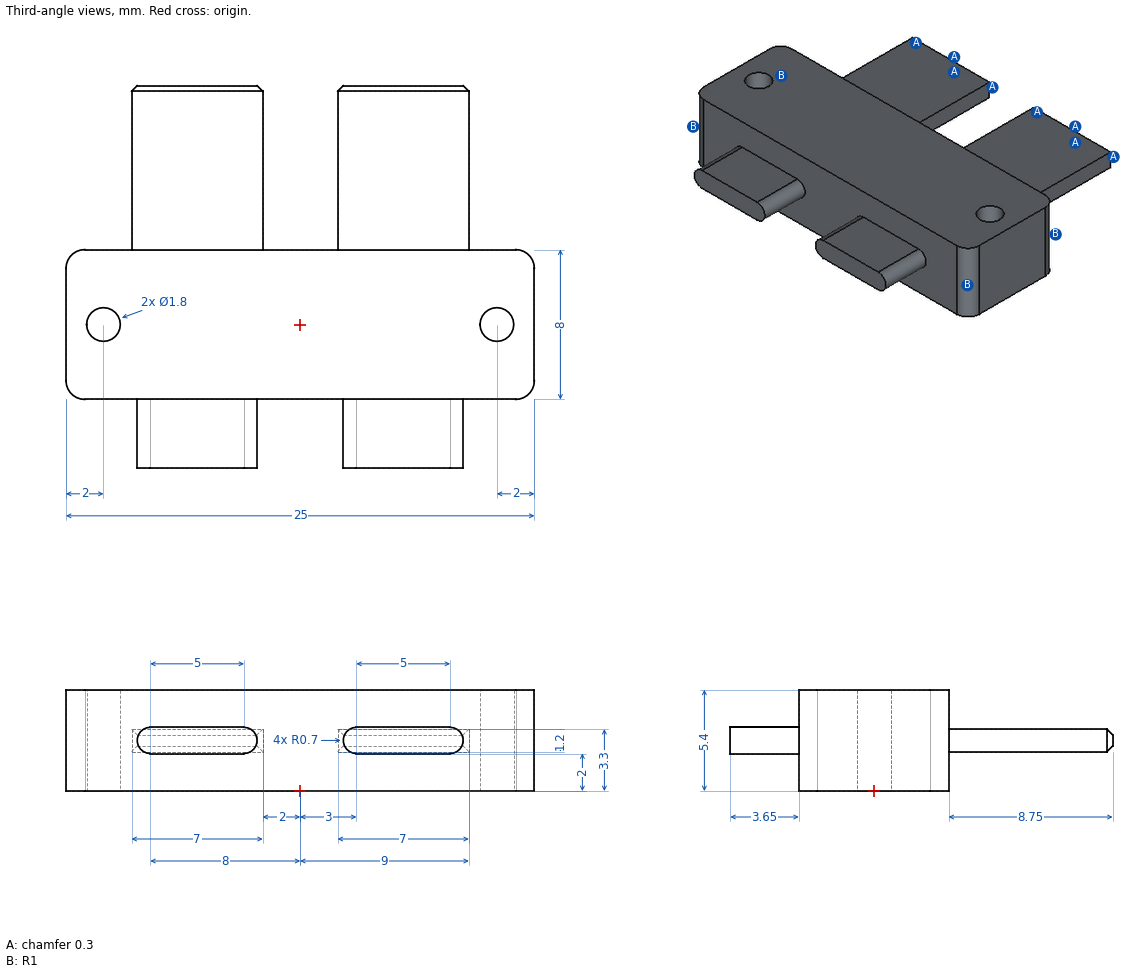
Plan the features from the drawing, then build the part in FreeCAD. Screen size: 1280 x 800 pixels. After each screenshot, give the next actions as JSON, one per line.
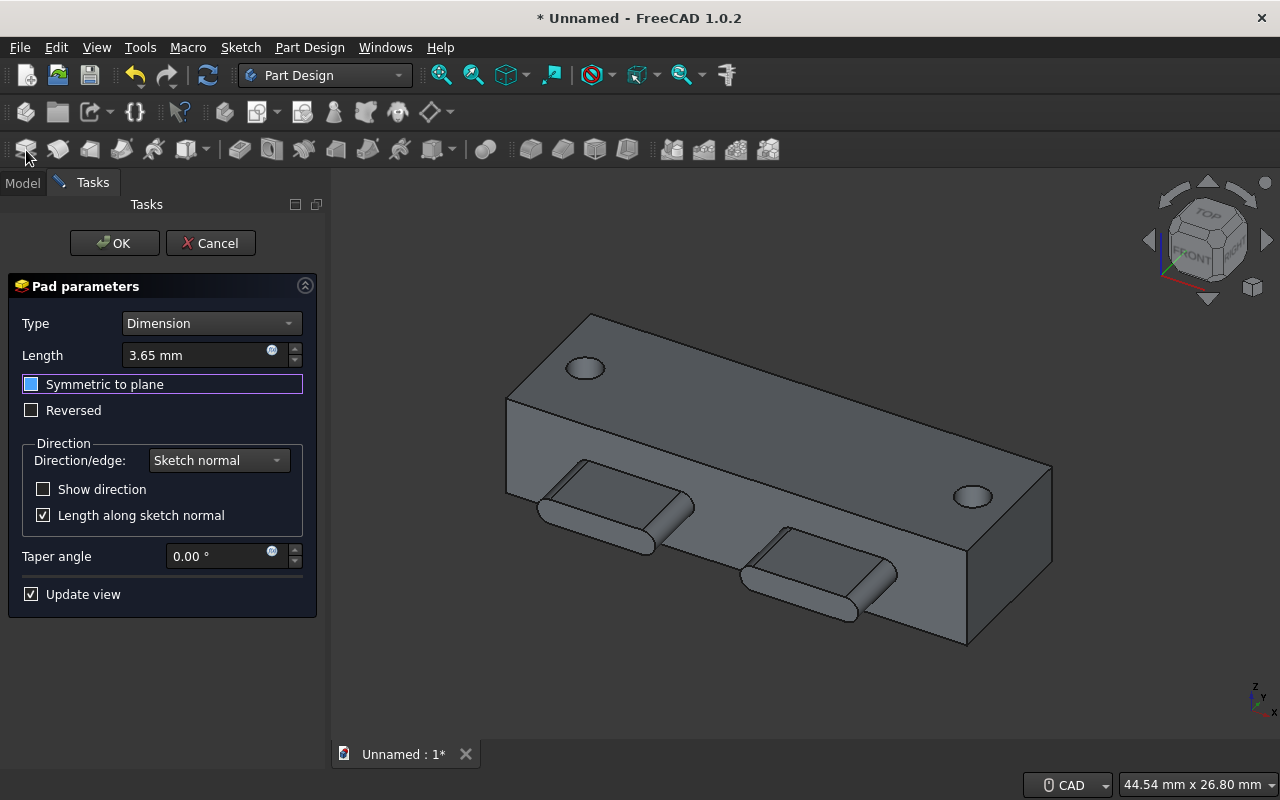
{"action": "left_click", "coordinate": [115, 243]}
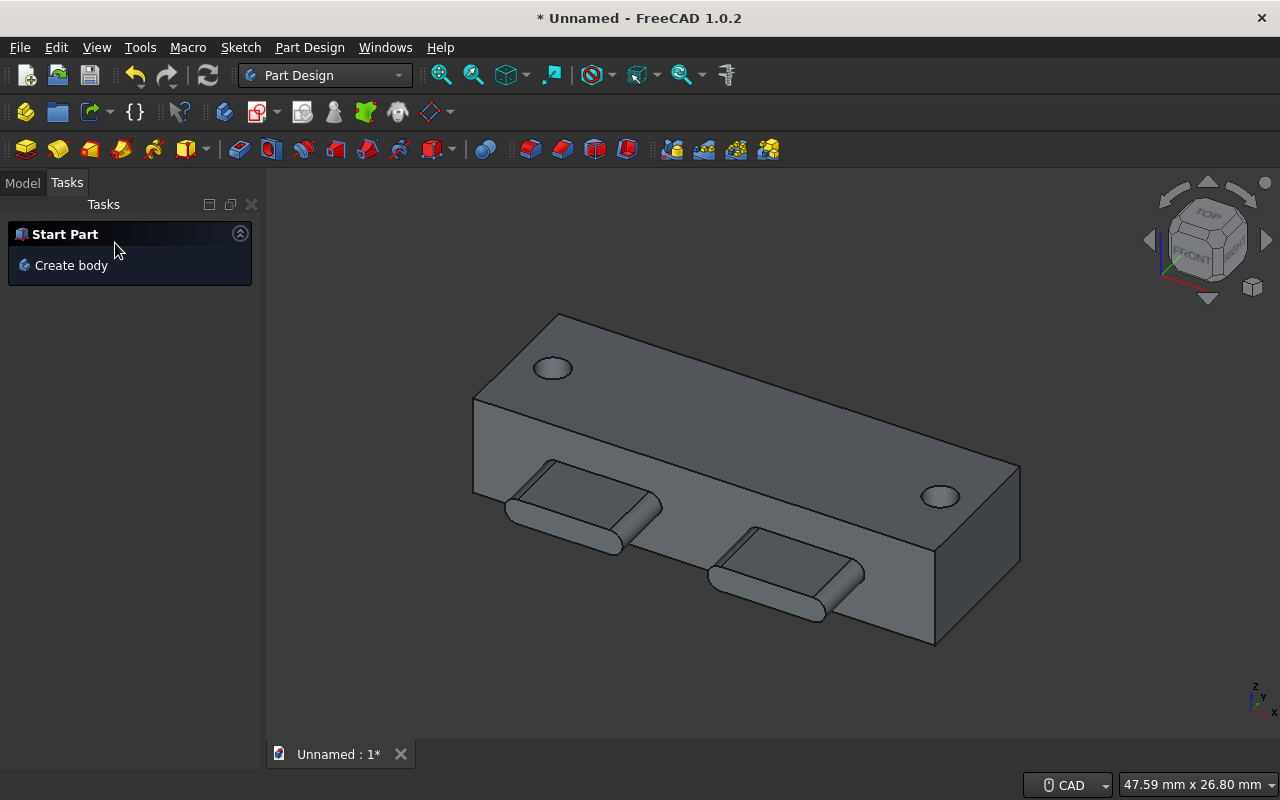
{"action": "key", "text": "4"}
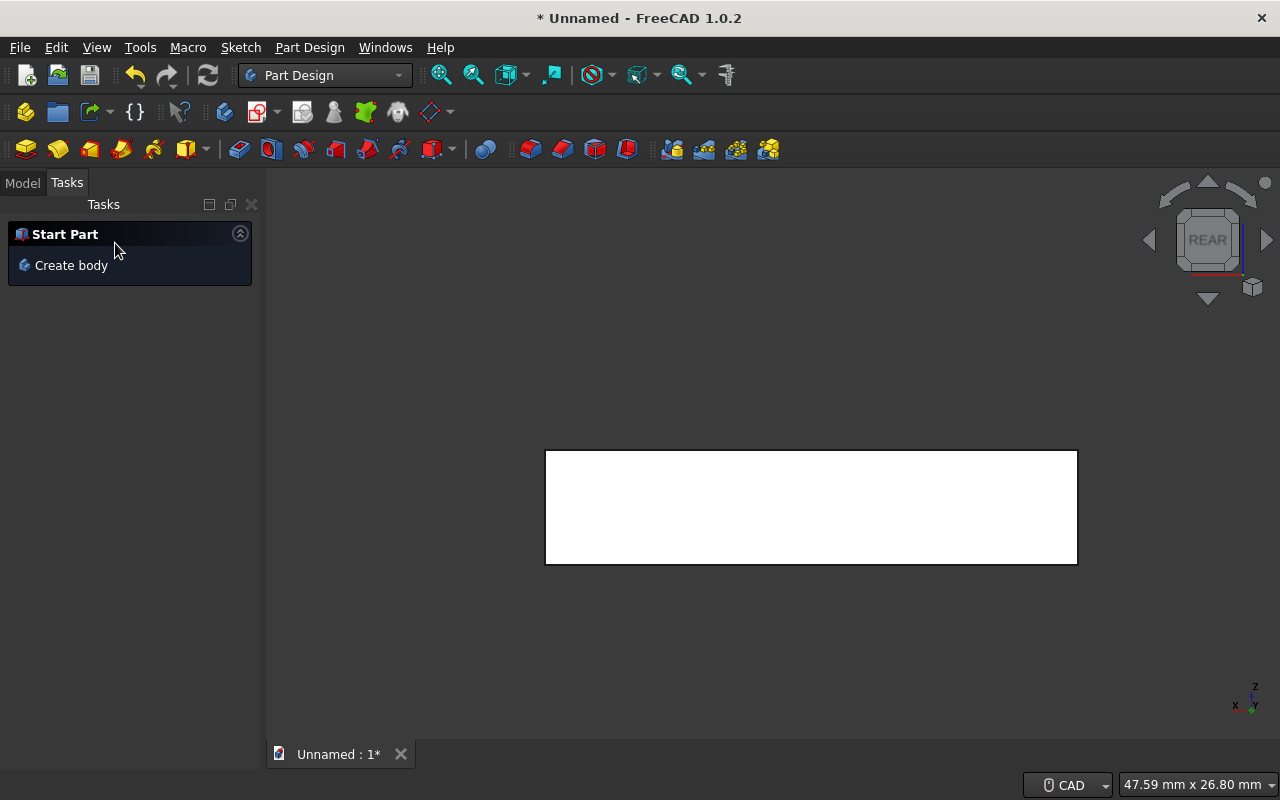
{"action": "left_click", "coordinate": [659, 506]}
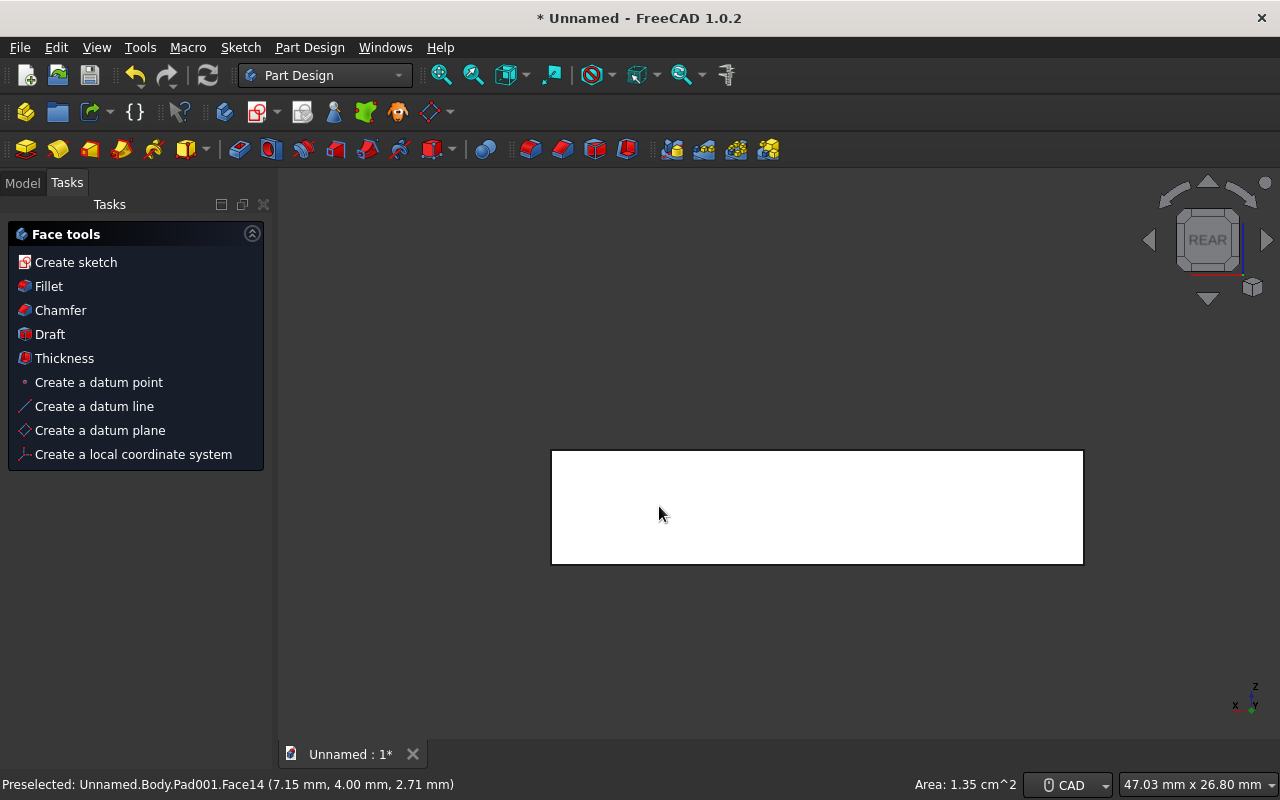
{"action": "left_click", "coordinate": [258, 112]}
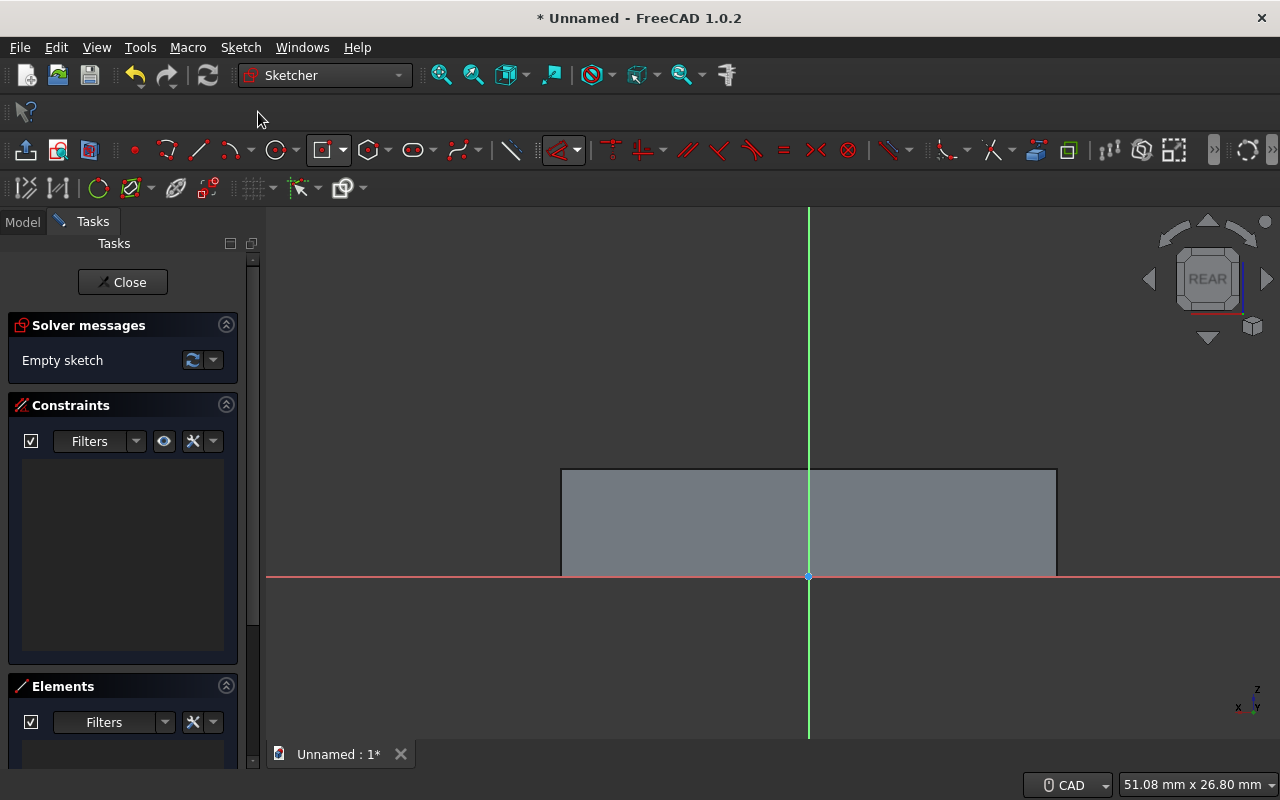
{"action": "scroll", "coordinate": [1020, 688], "scroll_direction": "up", "scroll_amount": 2}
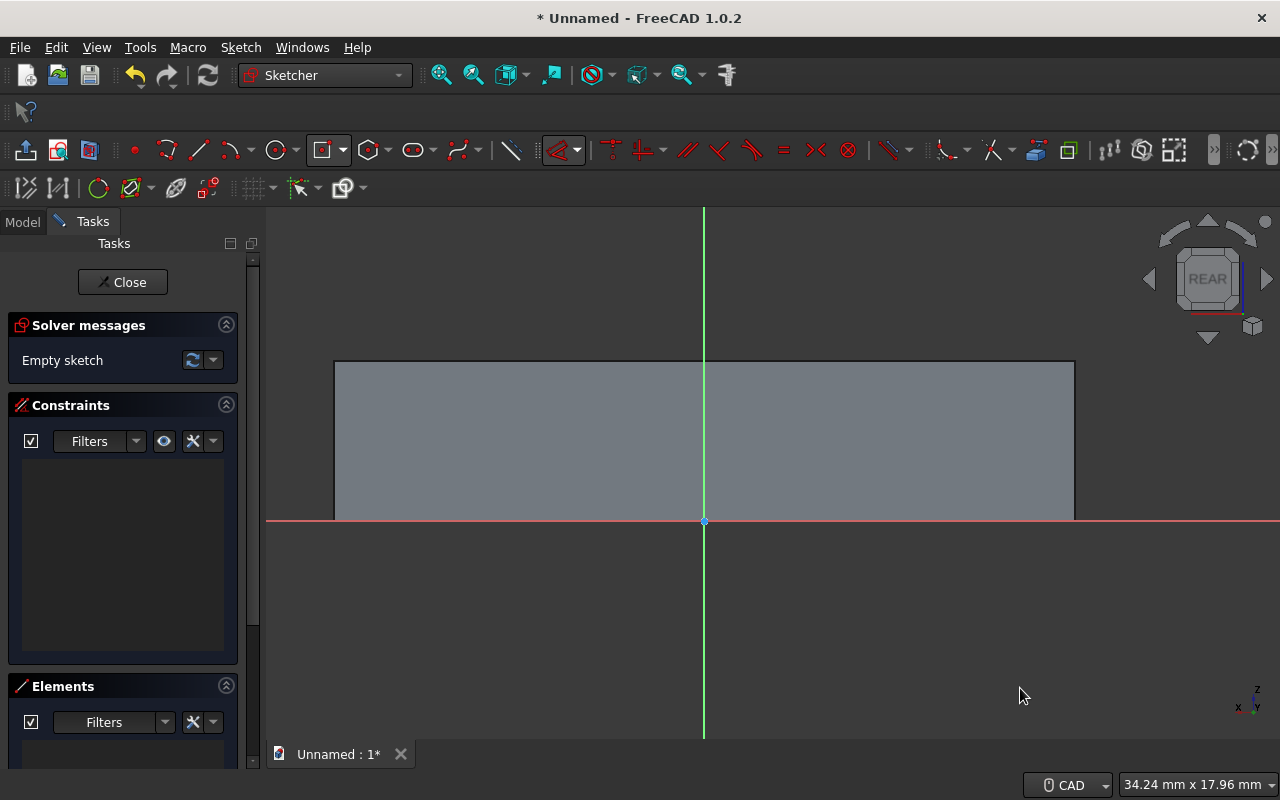
{"action": "key", "text": "g r"}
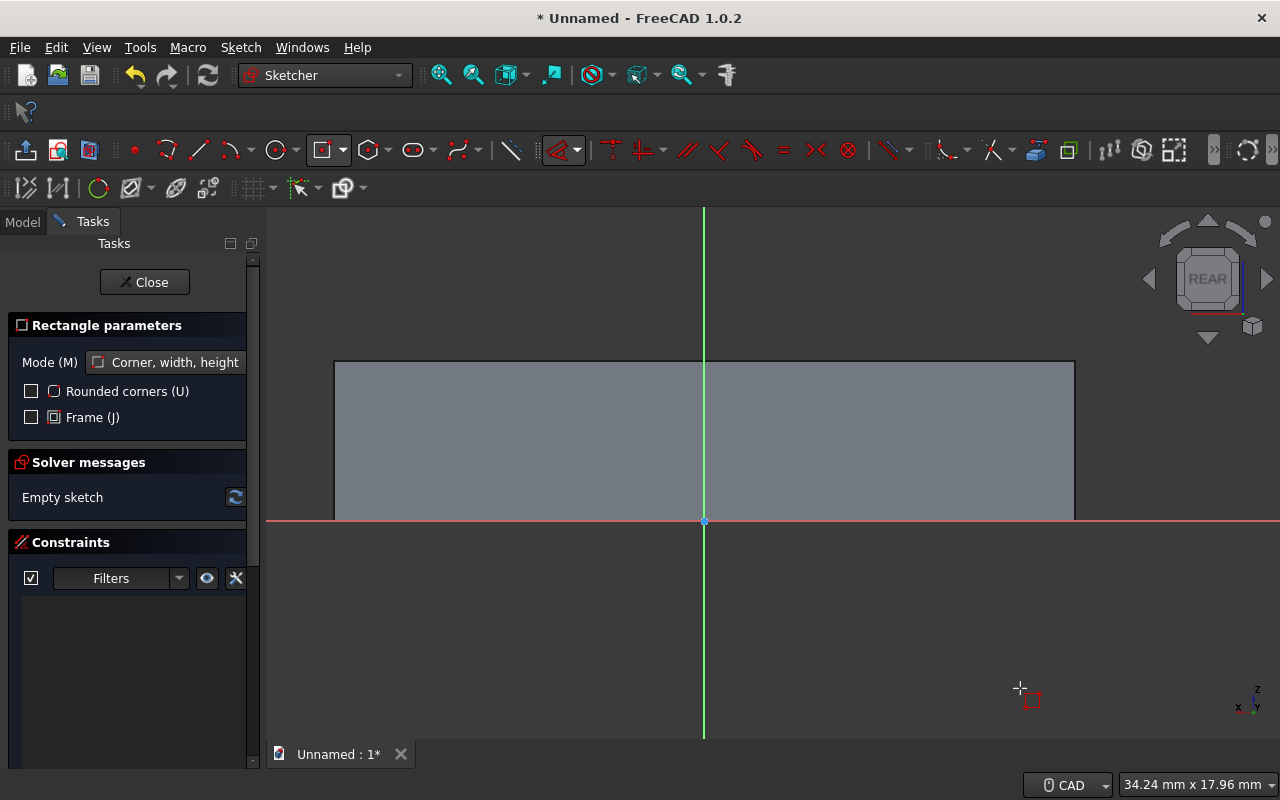
{"action": "left_click", "coordinate": [438, 424]}
{"action": "mouse_move", "coordinate": [645, 459]}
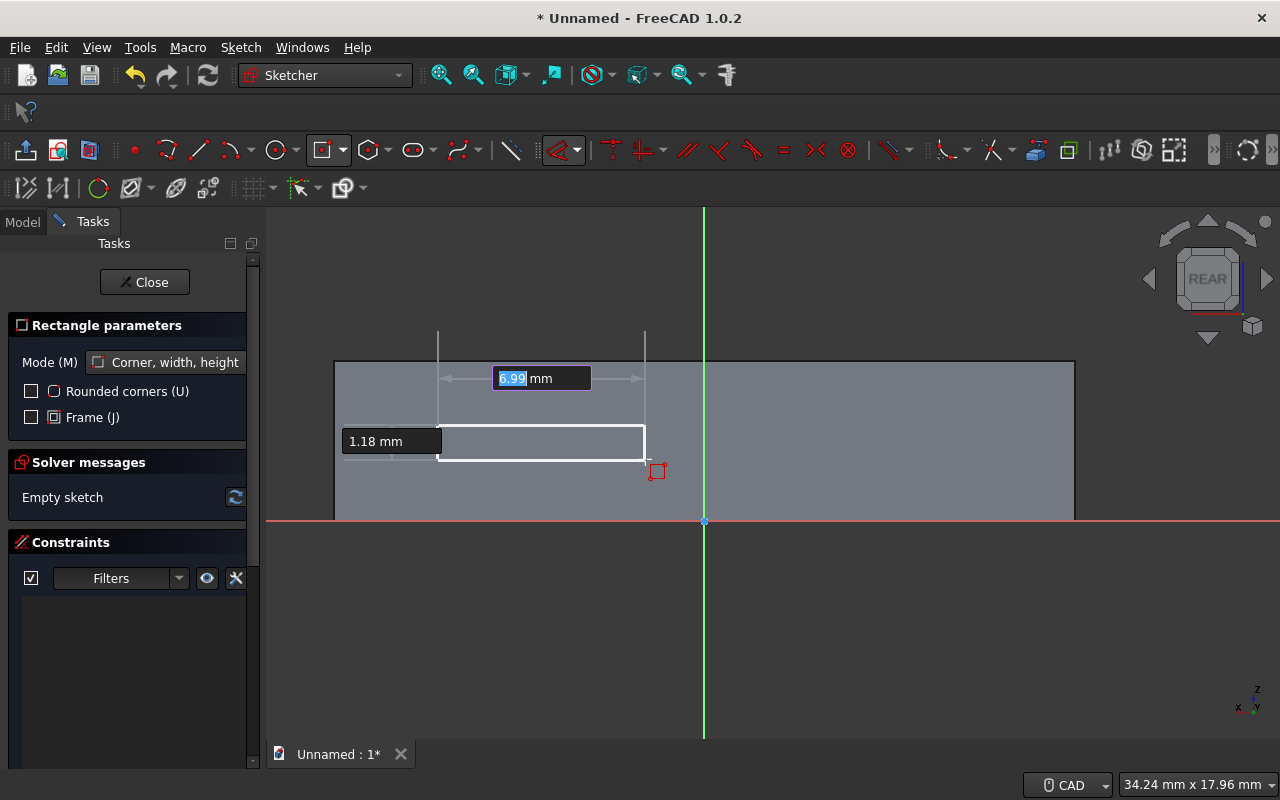
{"action": "type", "text": "7"}
{"action": "key", "text": "Tab"}
{"action": "type", "text": "1.2"}
{"action": "key", "text": "Return"}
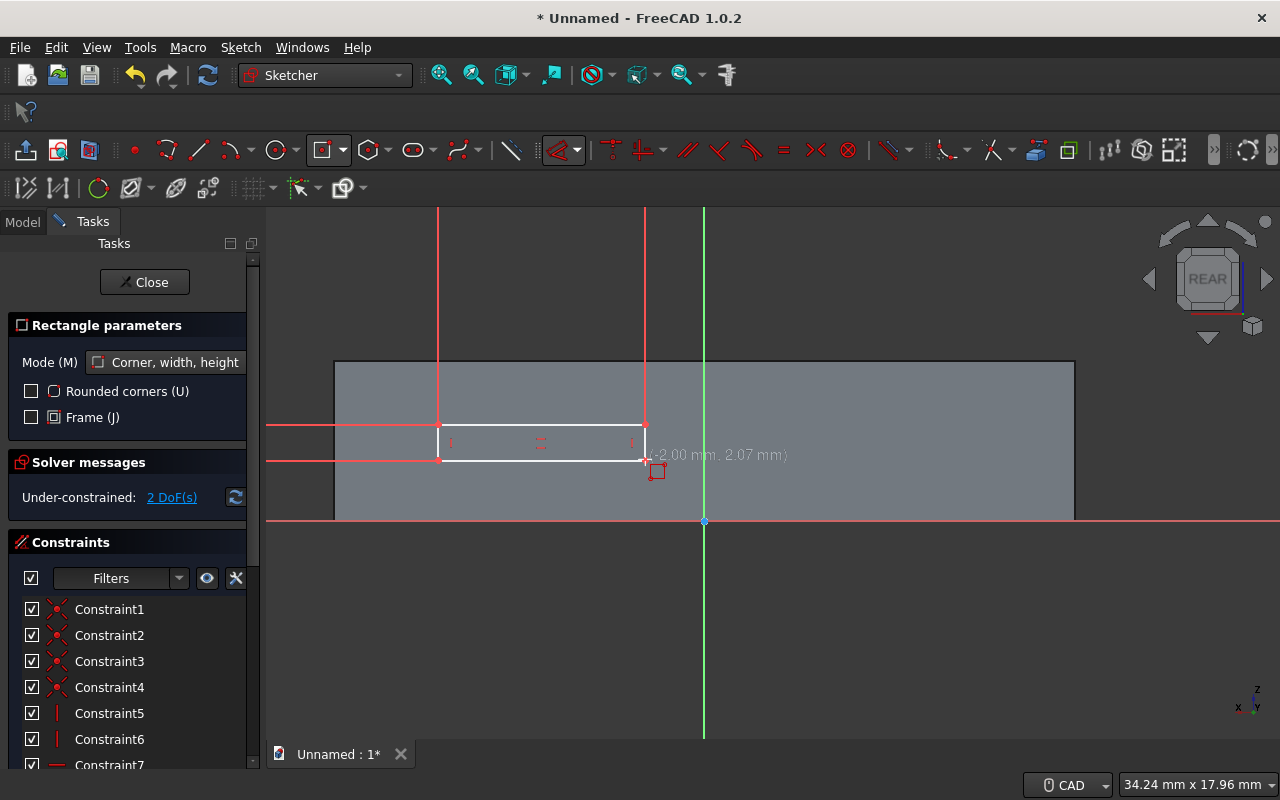
{"action": "left_click", "coordinate": [764, 424]}
{"action": "mouse_move", "coordinate": [971, 459]}